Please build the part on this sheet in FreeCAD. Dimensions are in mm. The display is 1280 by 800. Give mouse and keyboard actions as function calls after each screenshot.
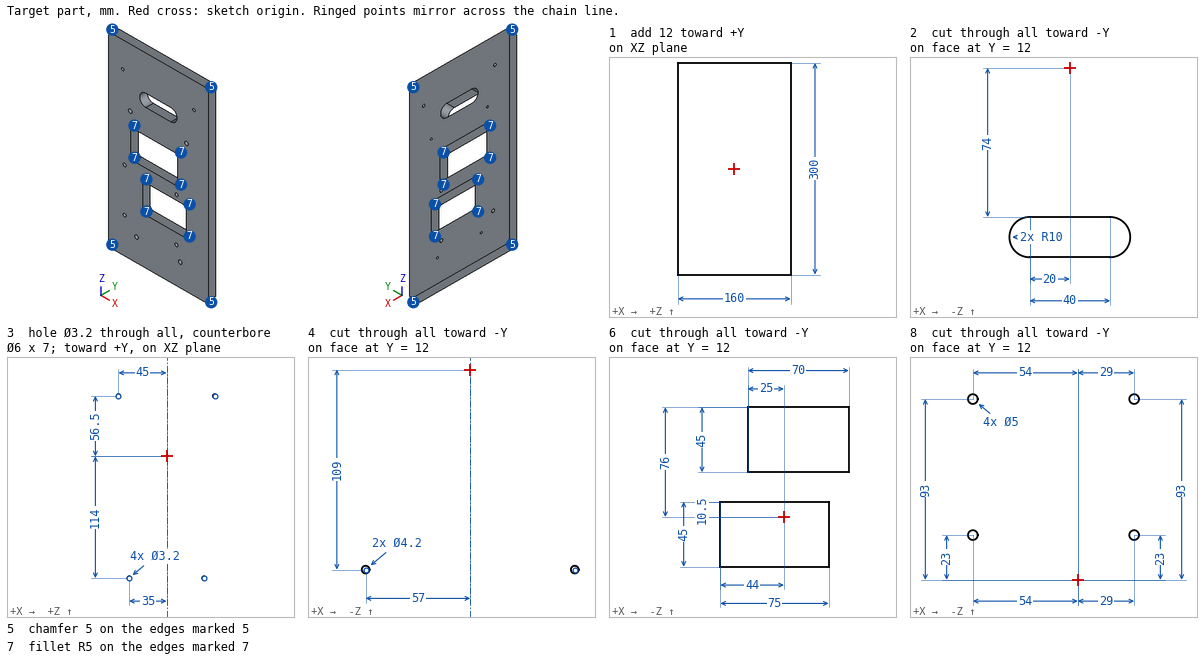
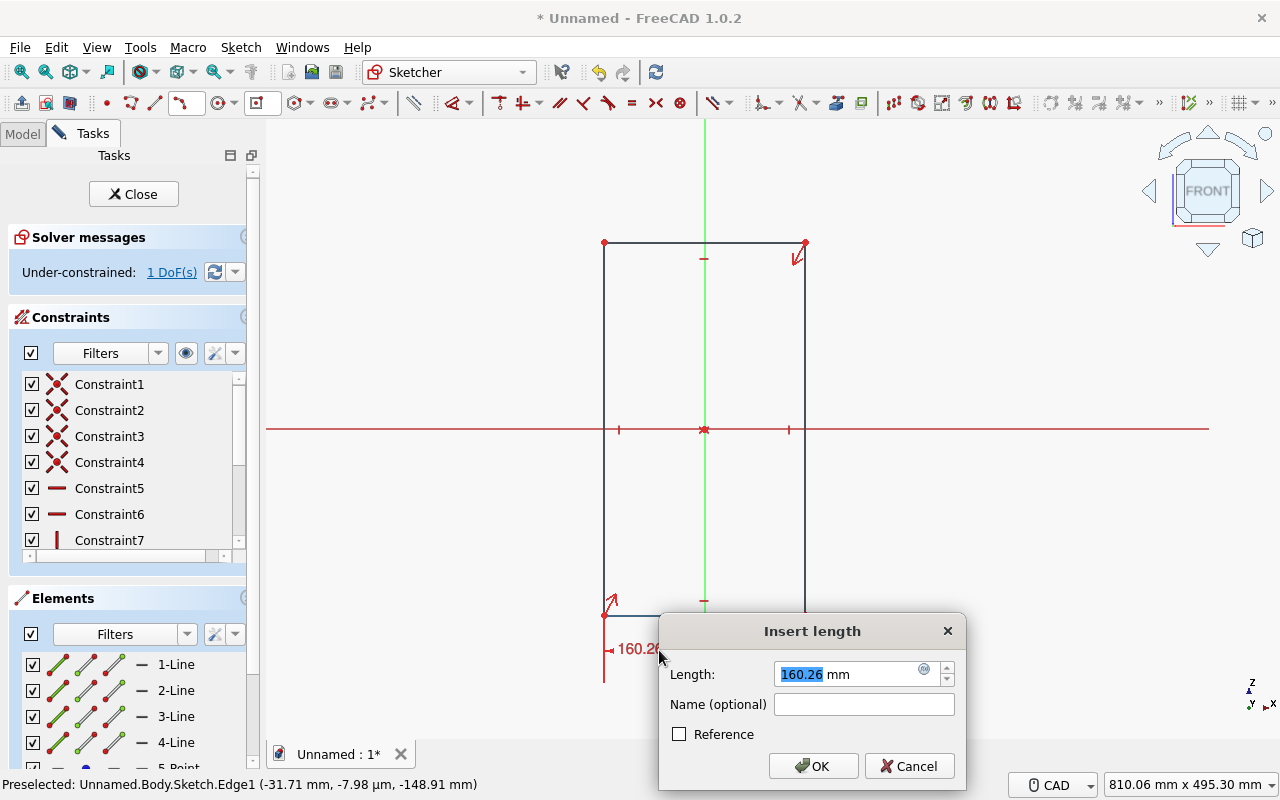
text(160)
key(Return)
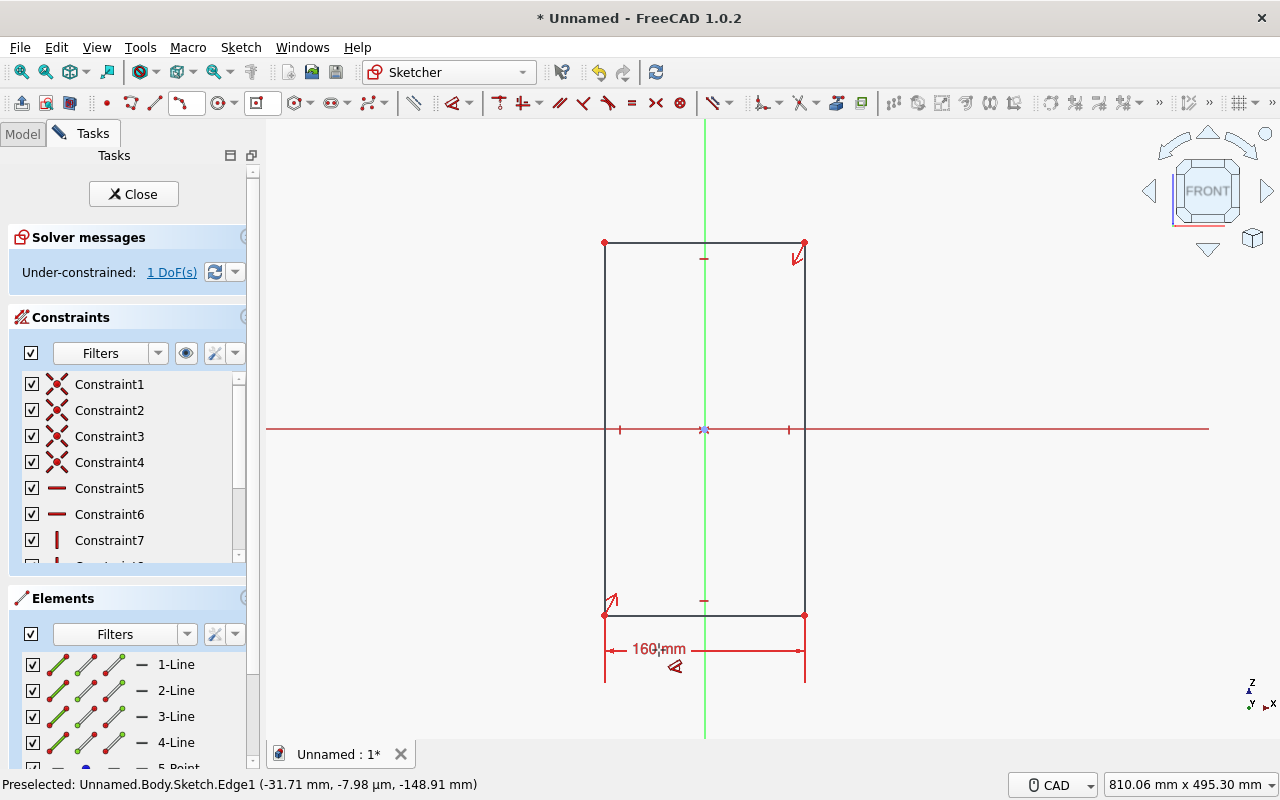
click(805, 504)
click(839, 344)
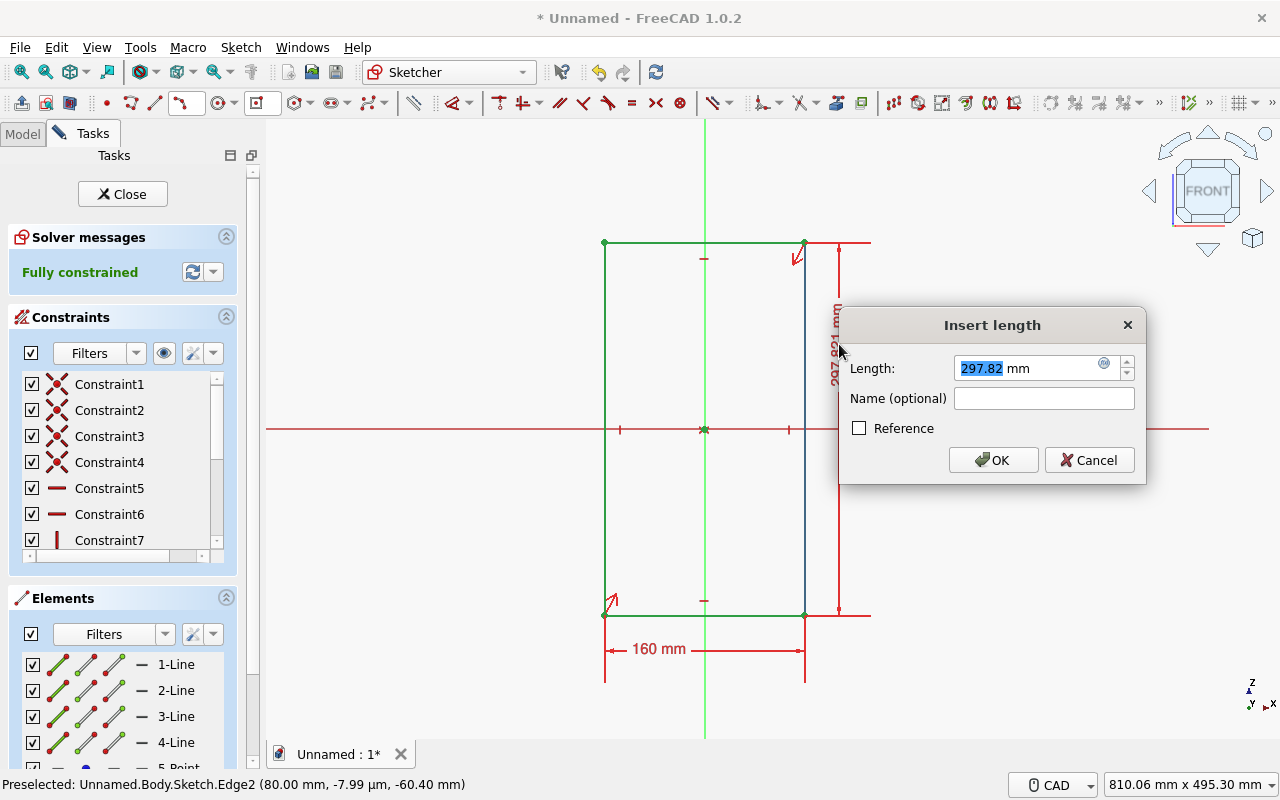
text(300)
key(Return)
key(Escape)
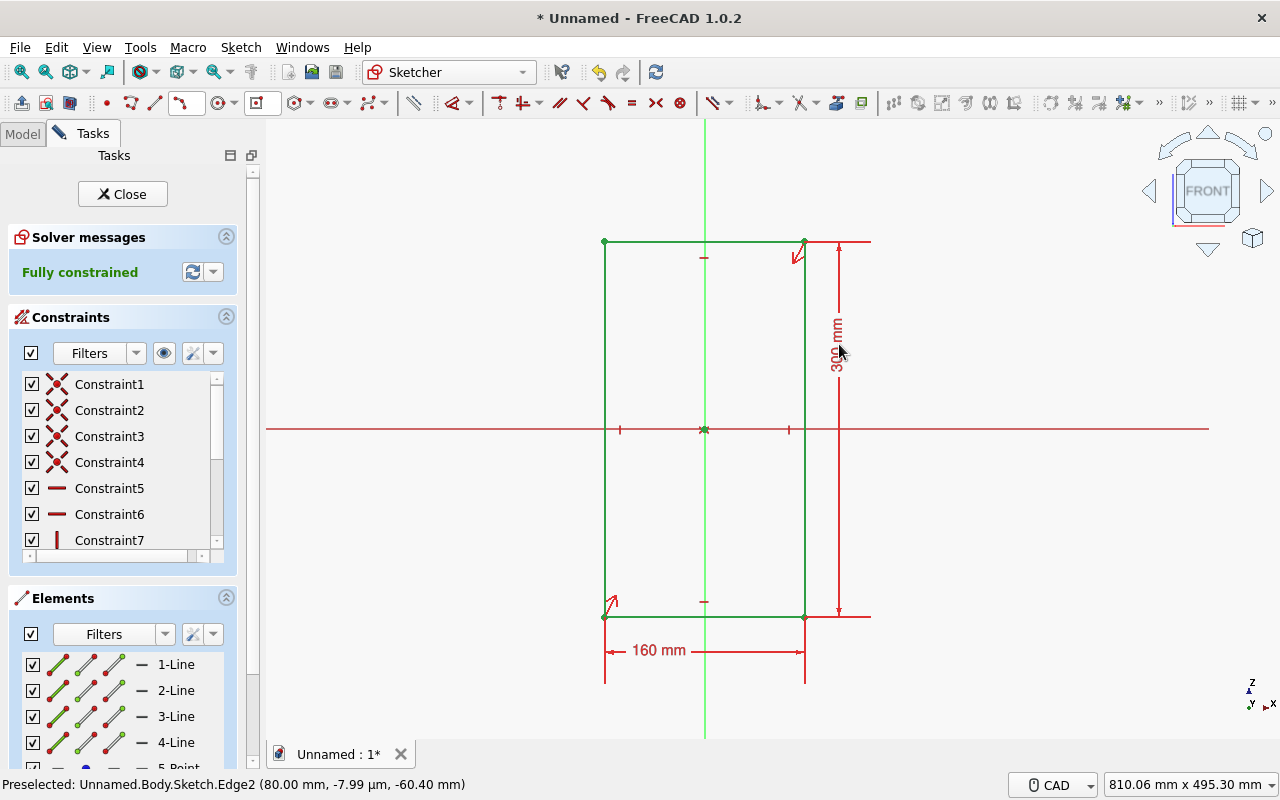
click(123, 194)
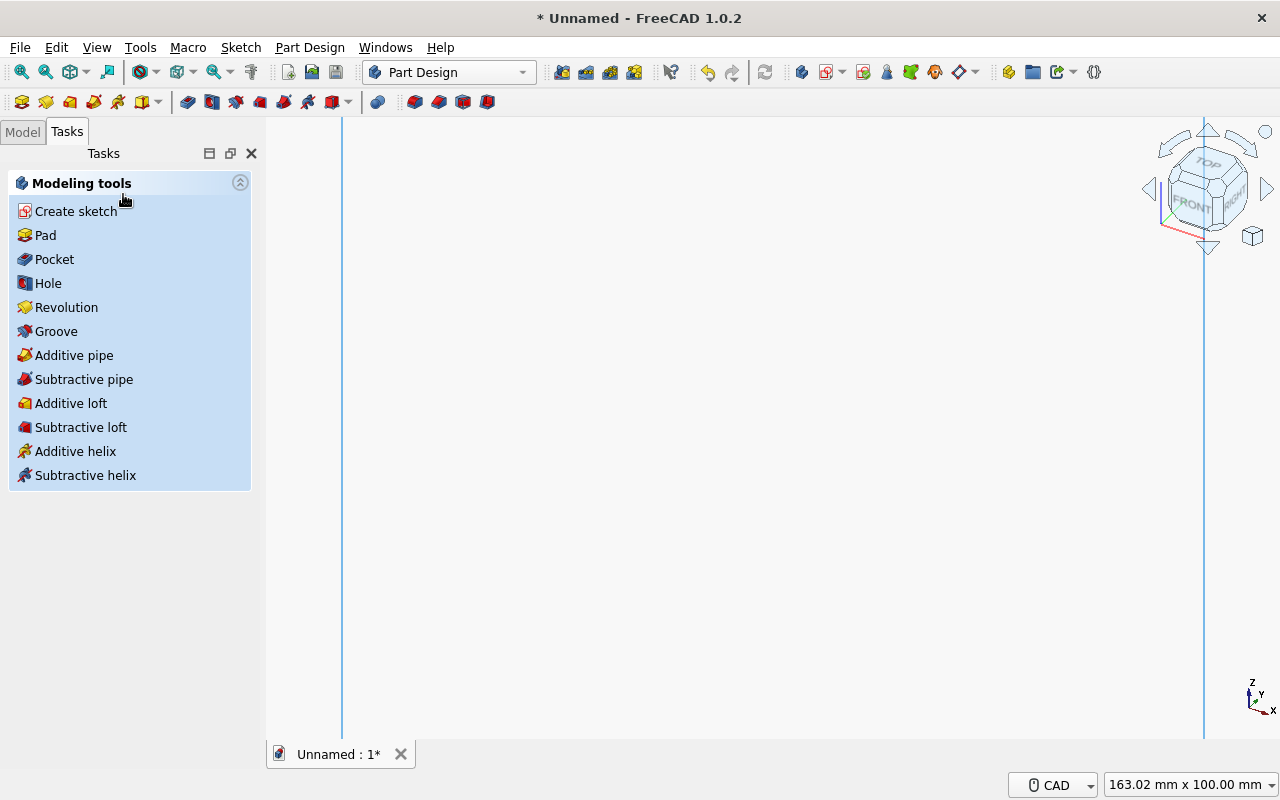
click(22, 102)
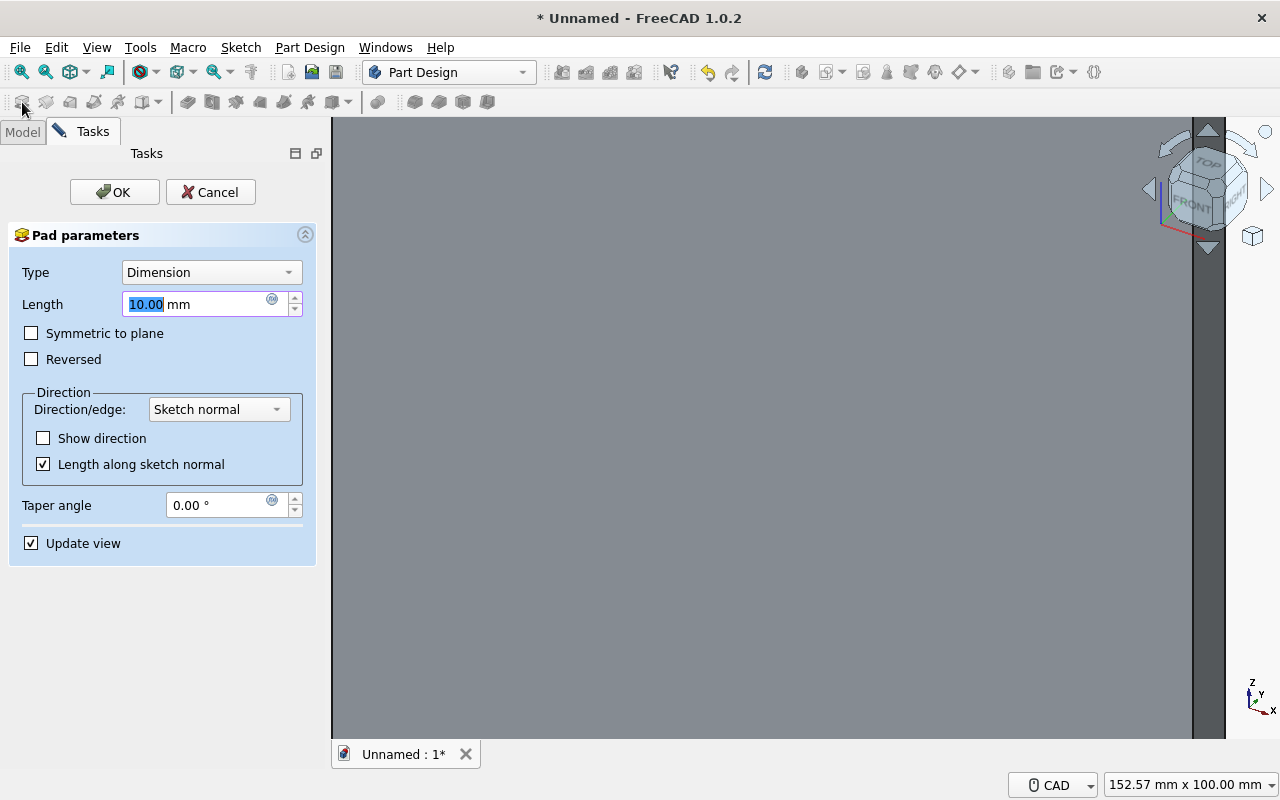
text(12)
key(Tab)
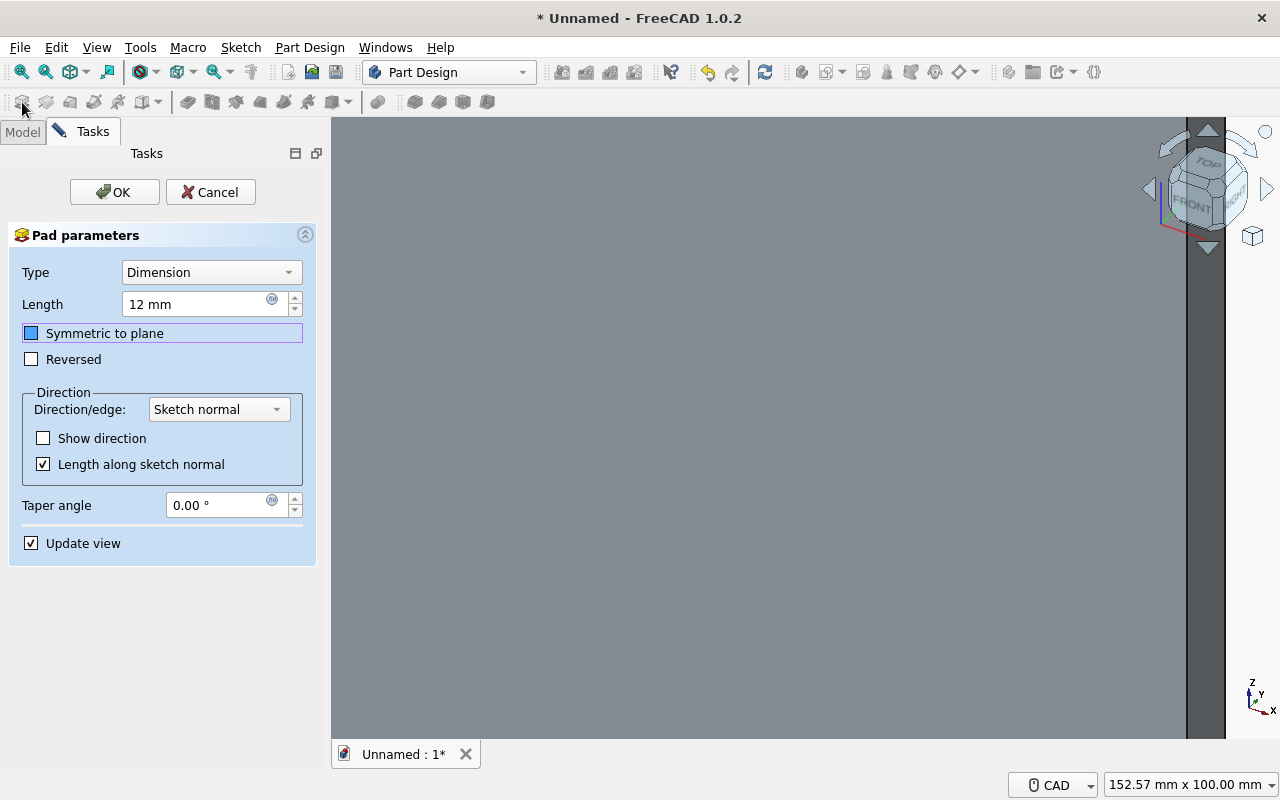
click(30, 359)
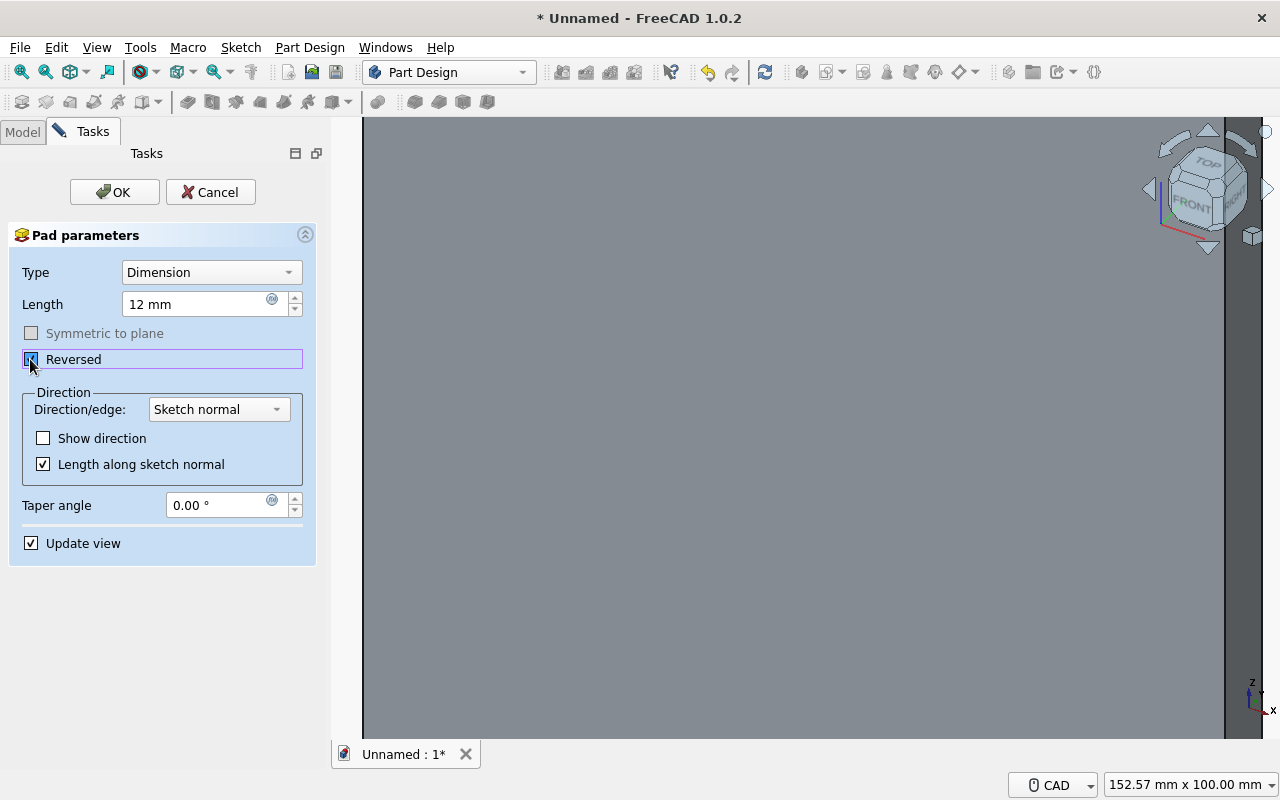
click(115, 192)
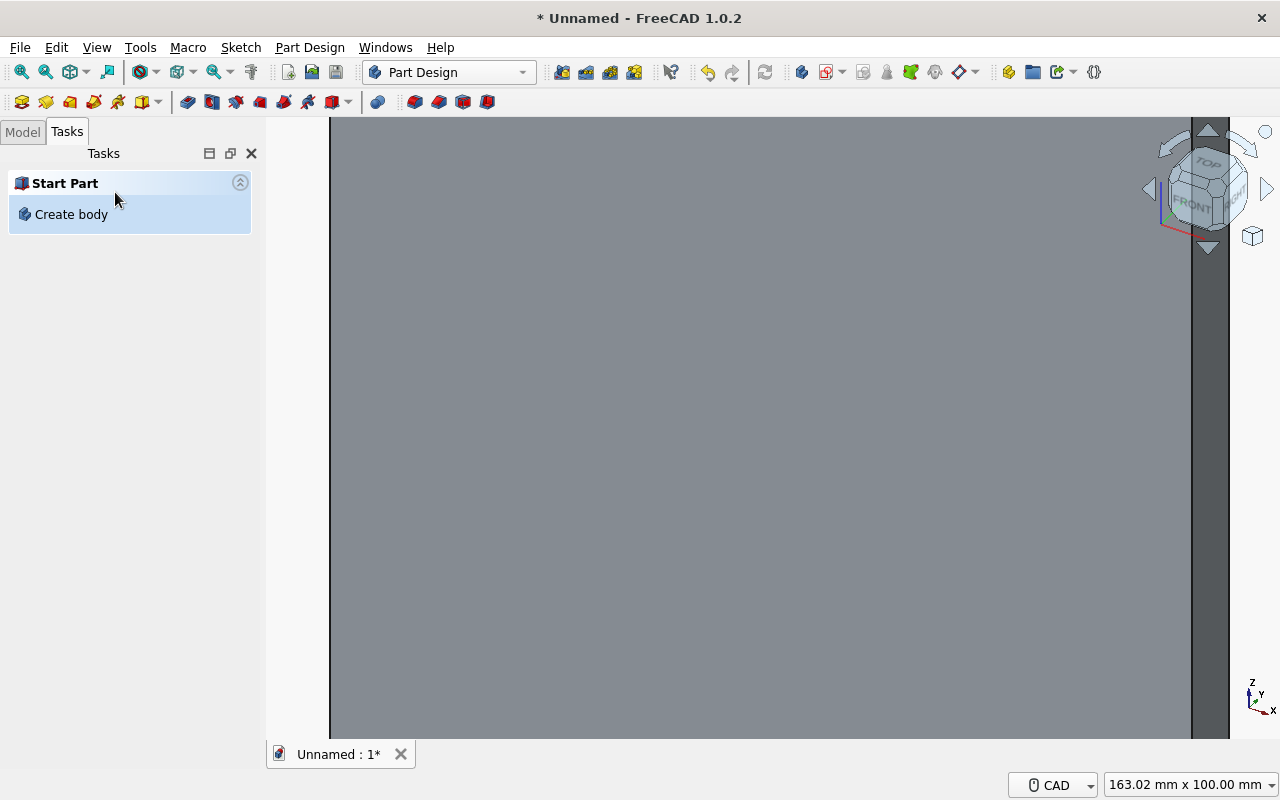
click(22, 72)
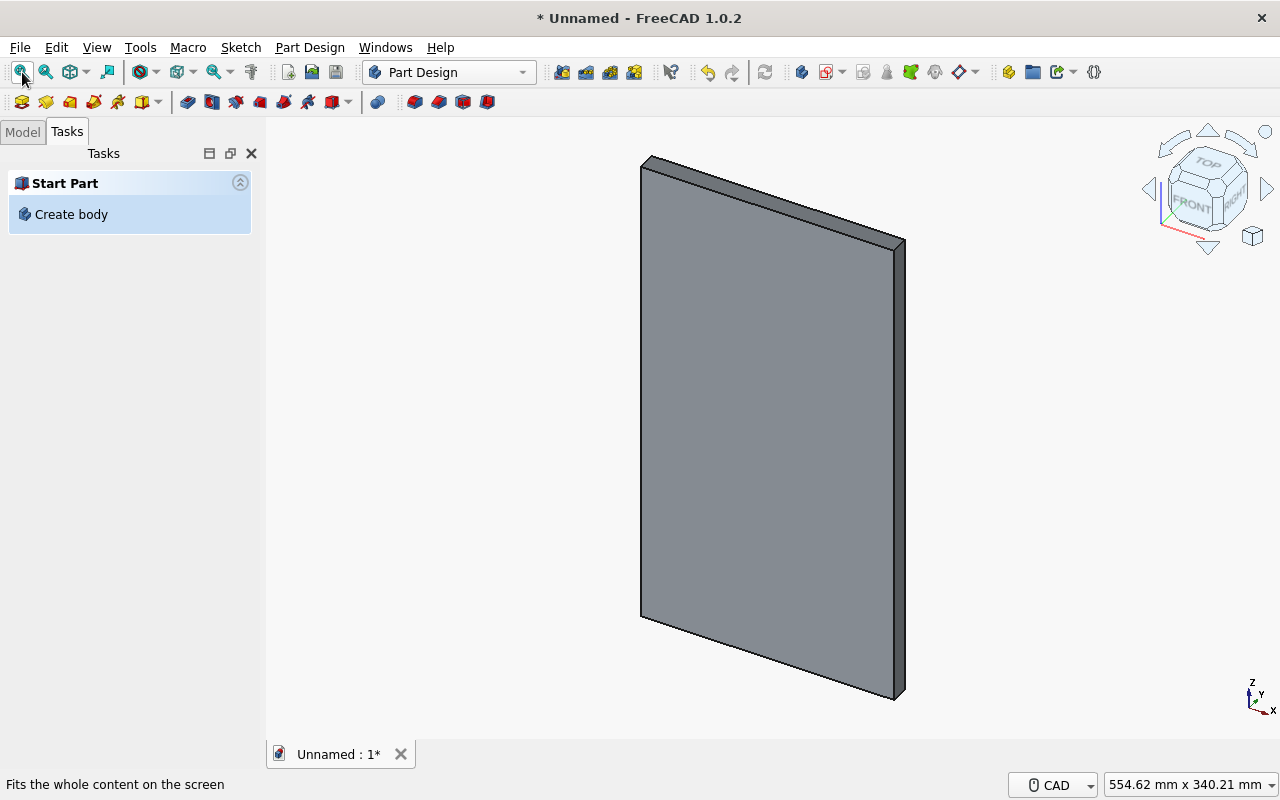
key(4)